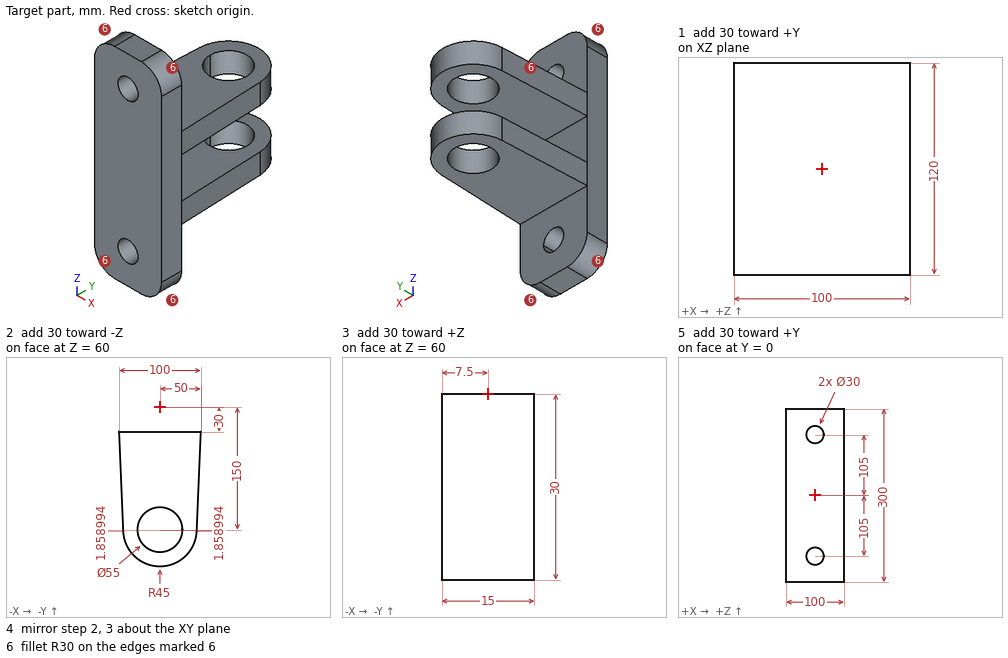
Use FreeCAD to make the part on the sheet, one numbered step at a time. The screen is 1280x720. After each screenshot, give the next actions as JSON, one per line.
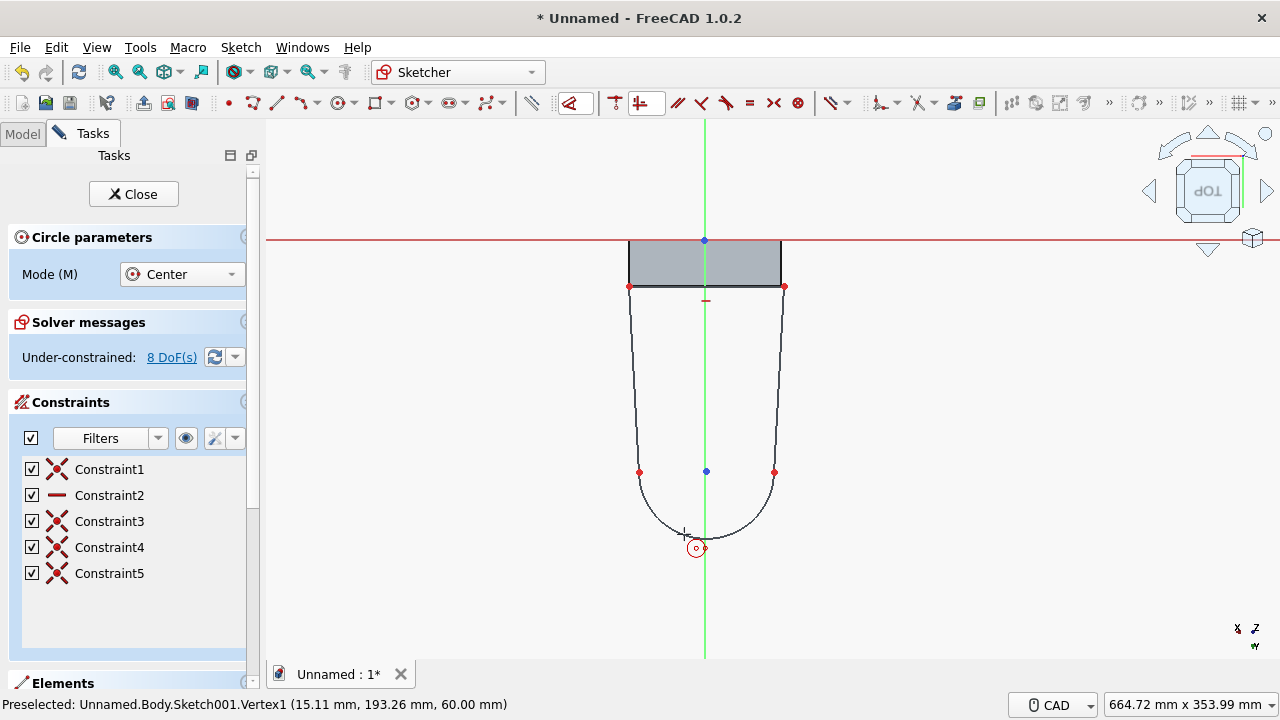
{"action": "left_click", "coordinate": [705, 469]}
{"action": "mouse_move", "coordinate": [735, 439]}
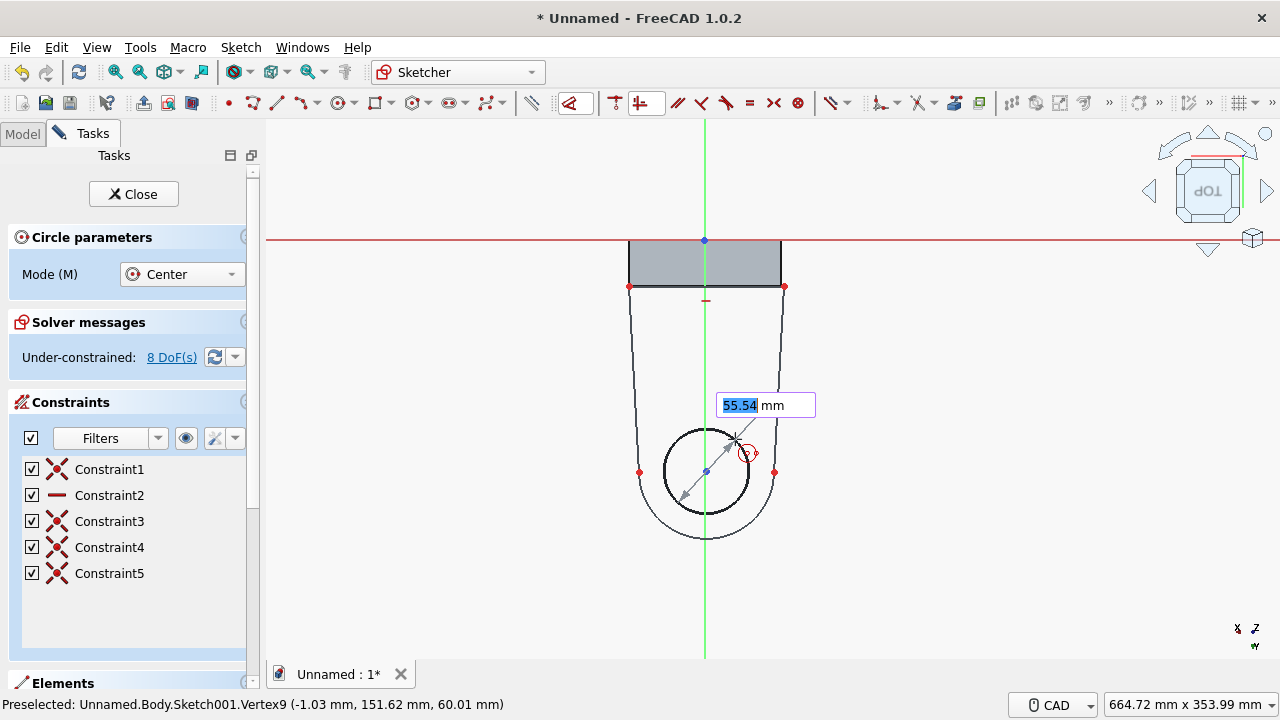
{"action": "type", "text": "55"}
{"action": "key", "text": "Return"}
{"action": "key", "text": "Escape"}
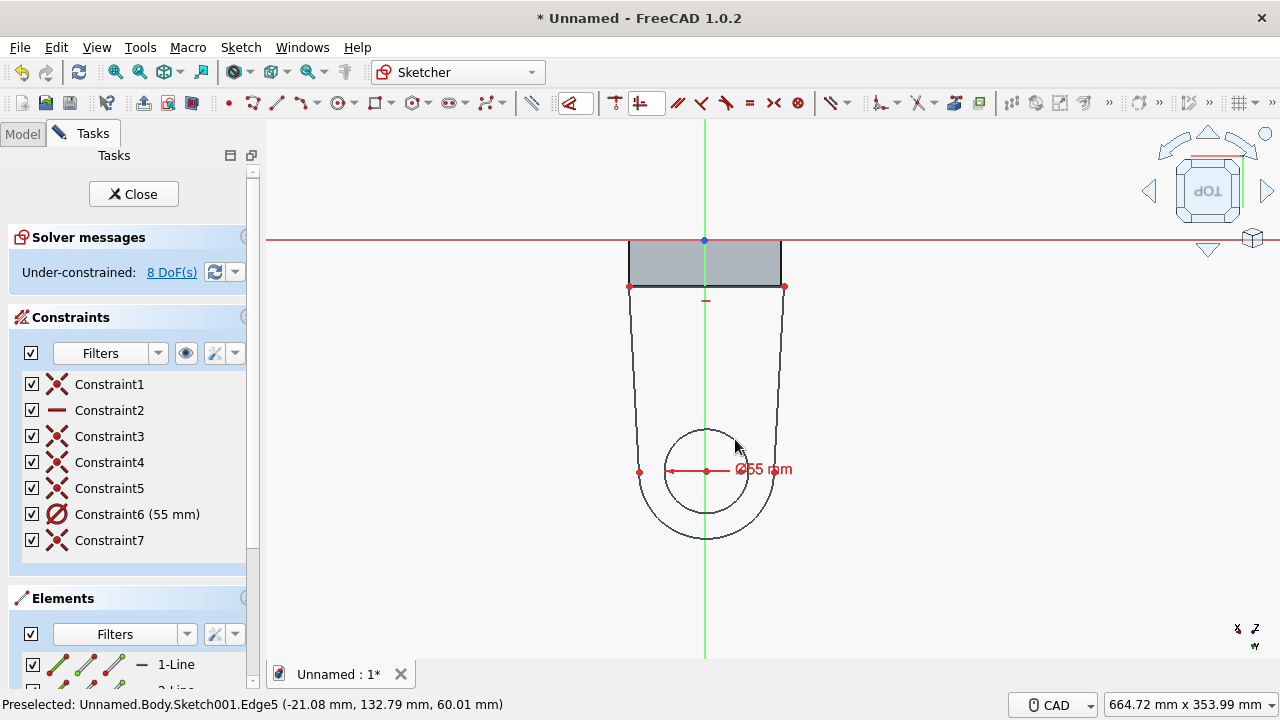
{"action": "left_click", "coordinate": [707, 471]}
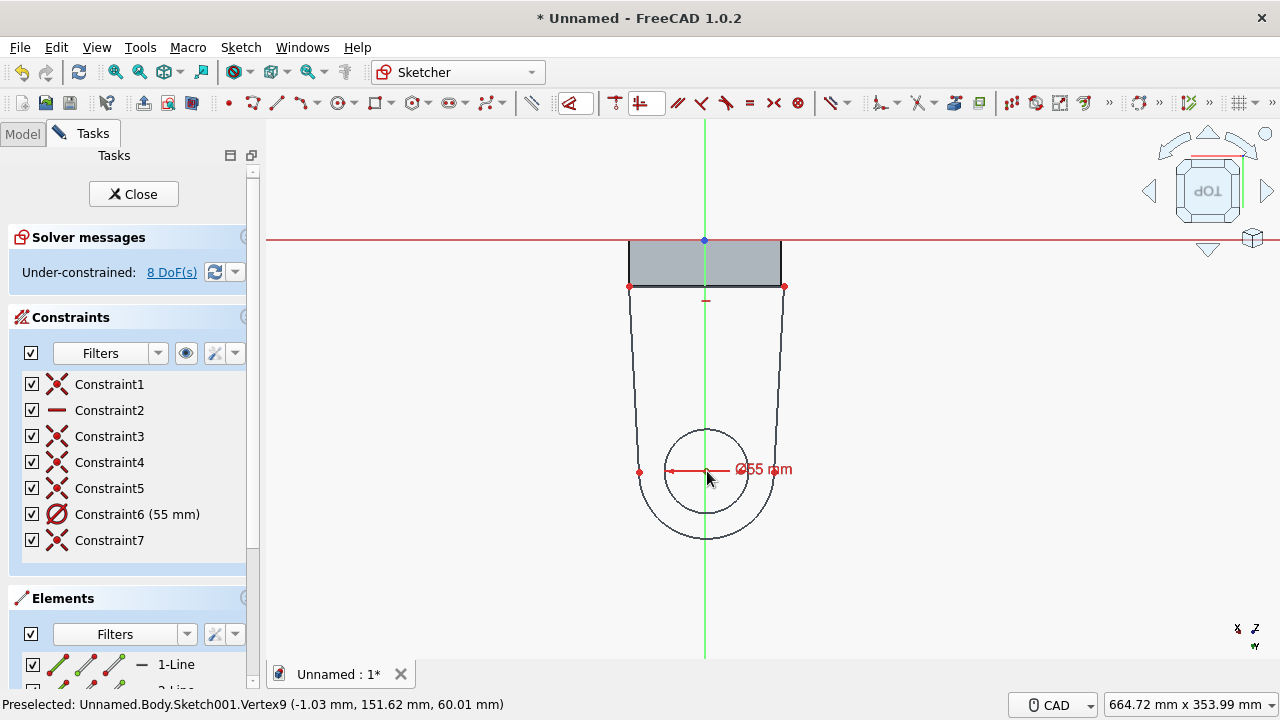
{"action": "left_click", "coordinate": [705, 596]}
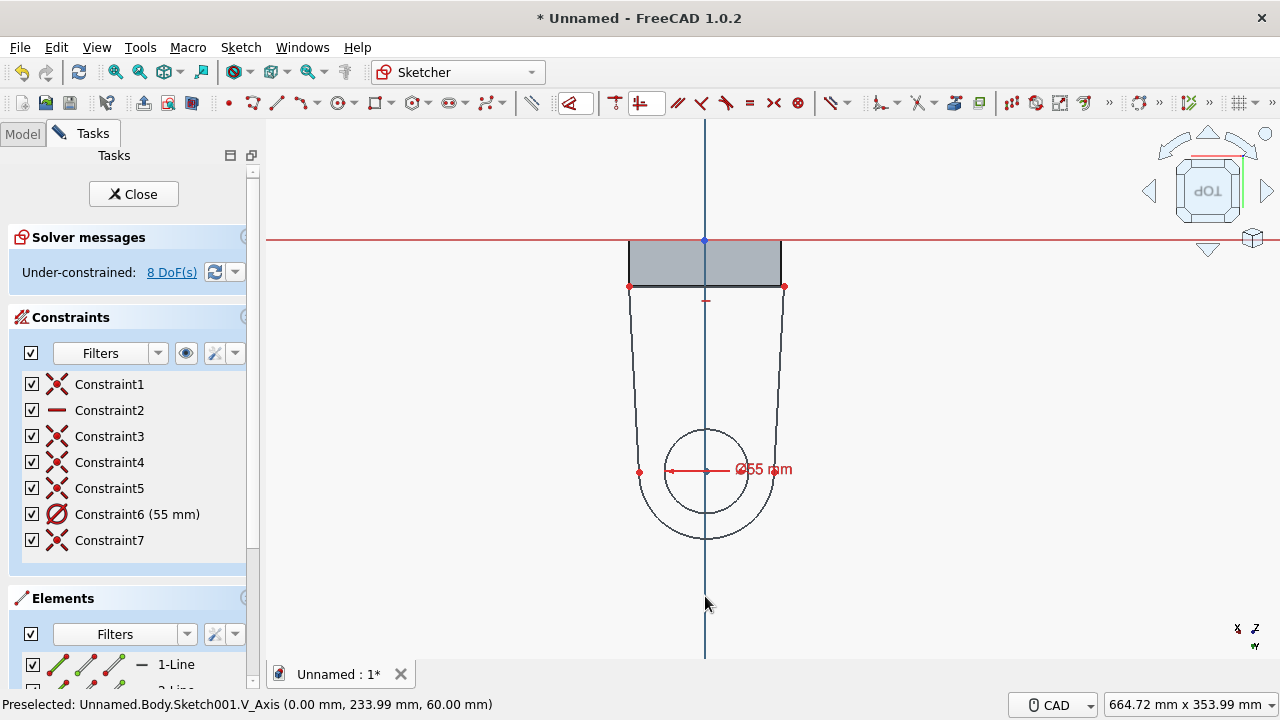
{"action": "key", "text": "c"}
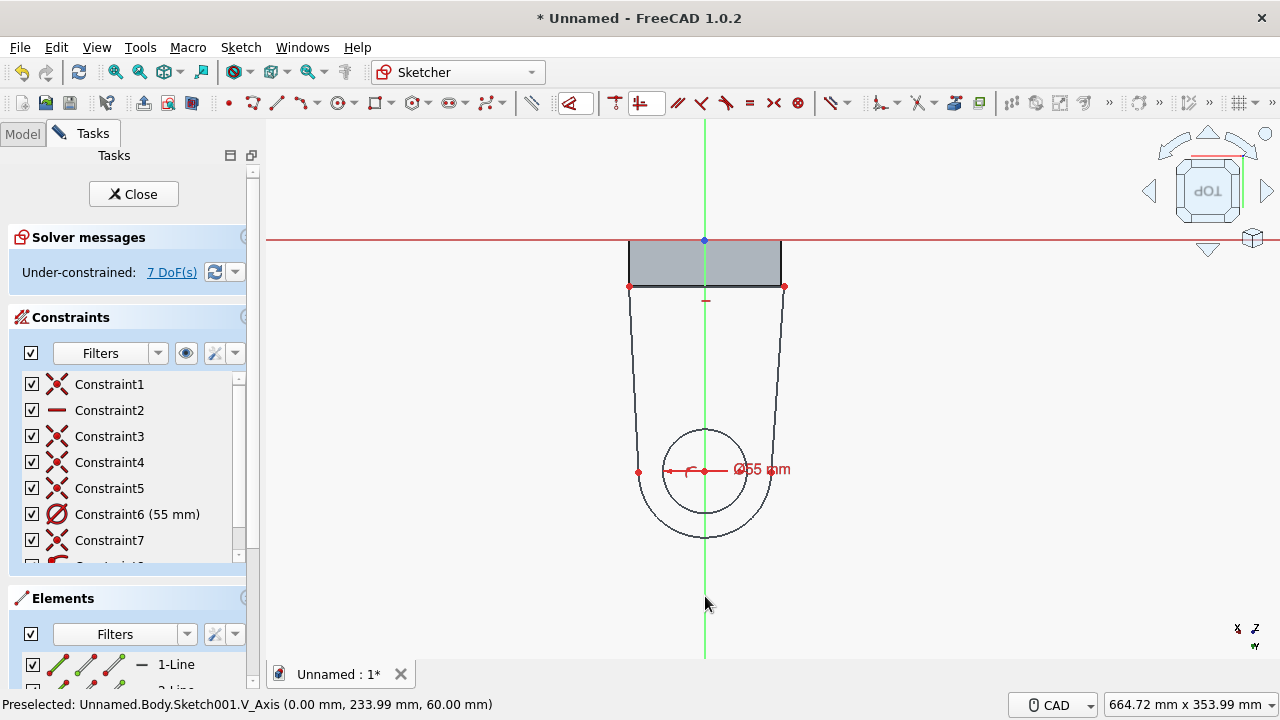
{"action": "left_click", "coordinate": [666, 525]}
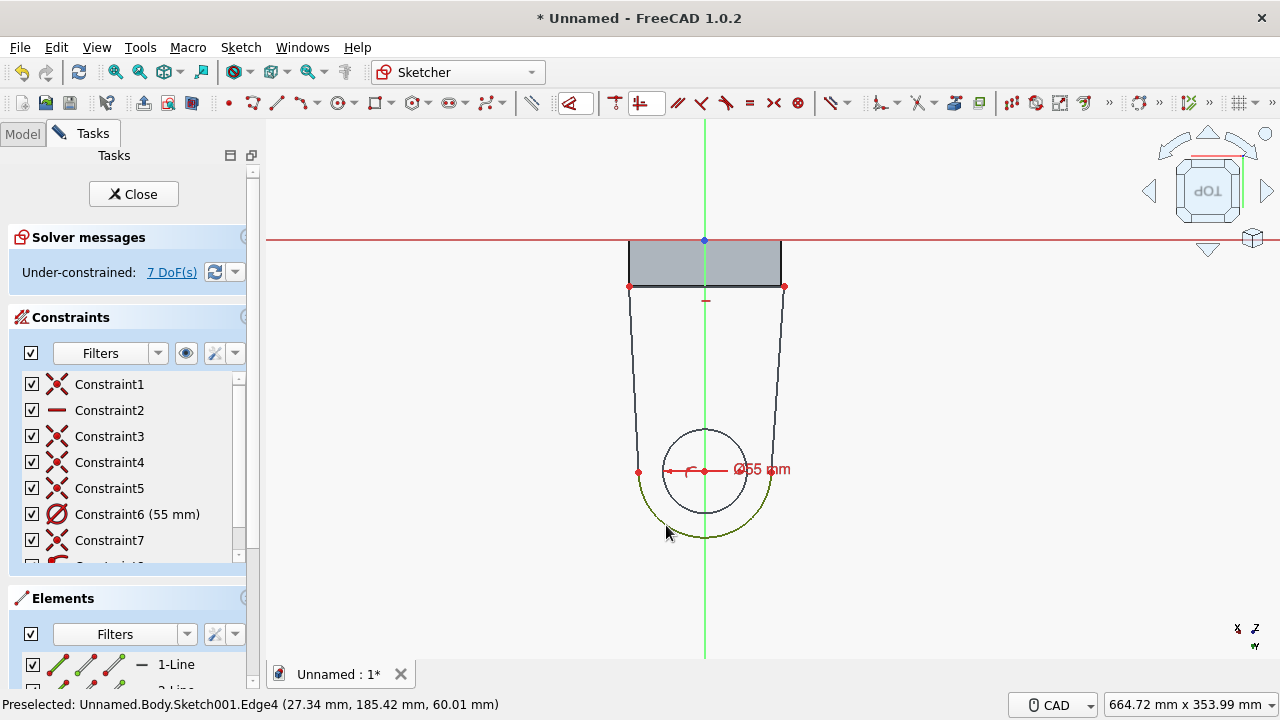
{"action": "key", "text": "k r"}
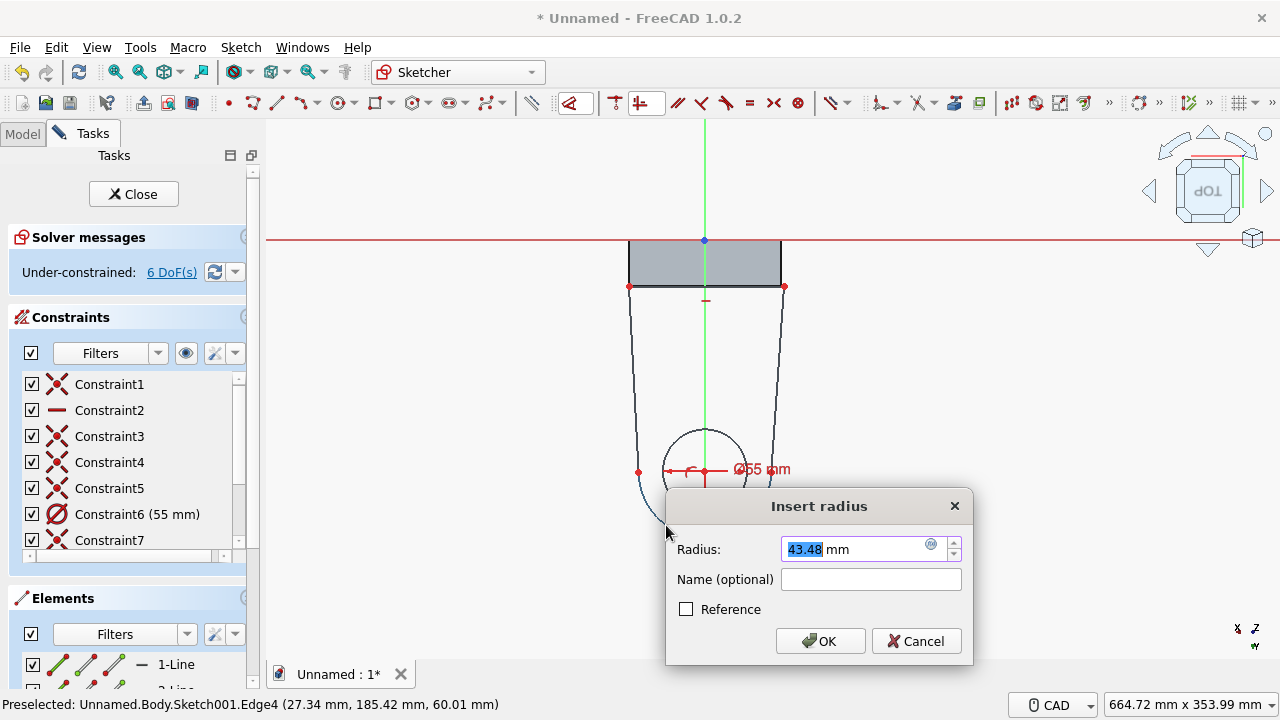
{"action": "type", "text": "45"}
{"action": "key", "text": "Return"}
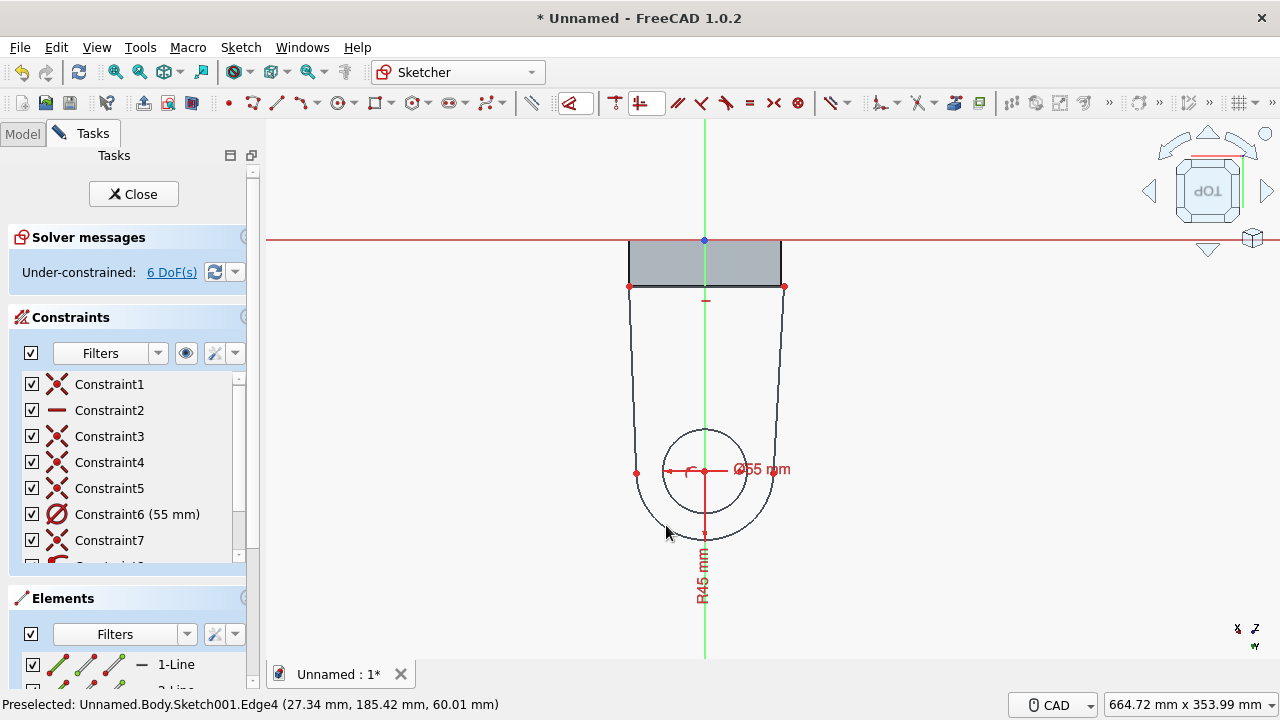
{"action": "left_click", "coordinate": [737, 287]}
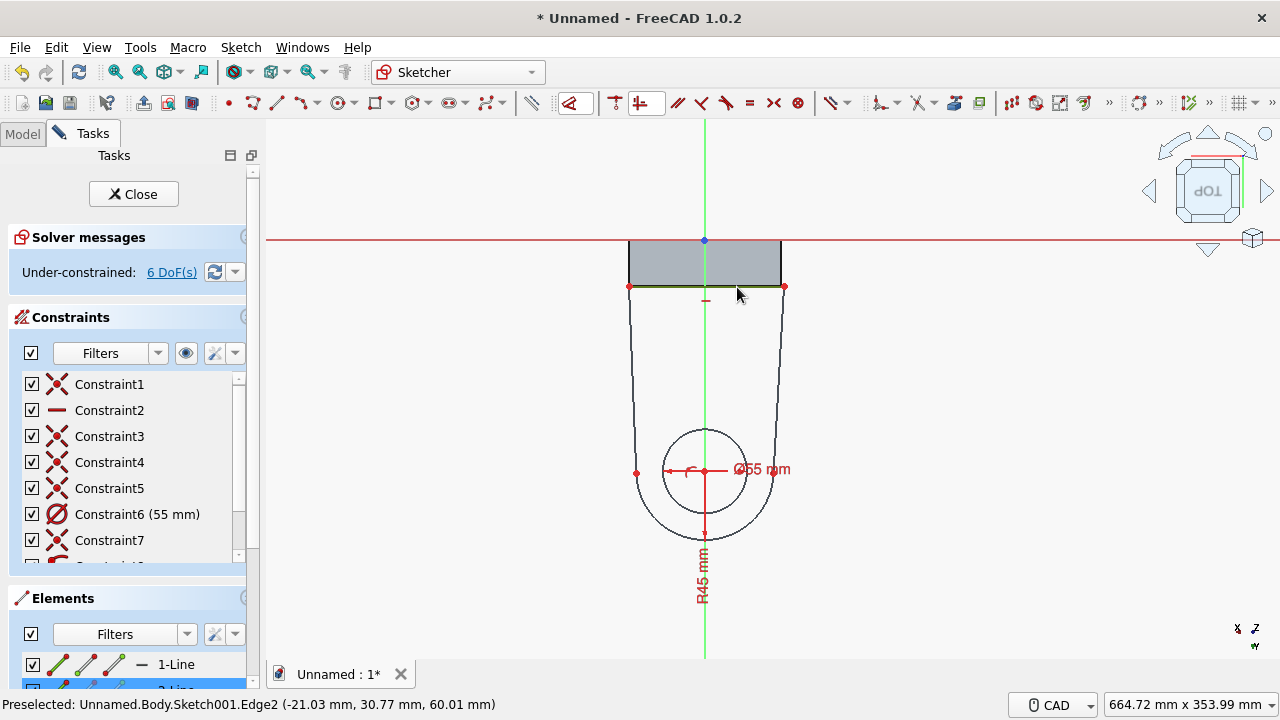
{"action": "key", "text": "l"}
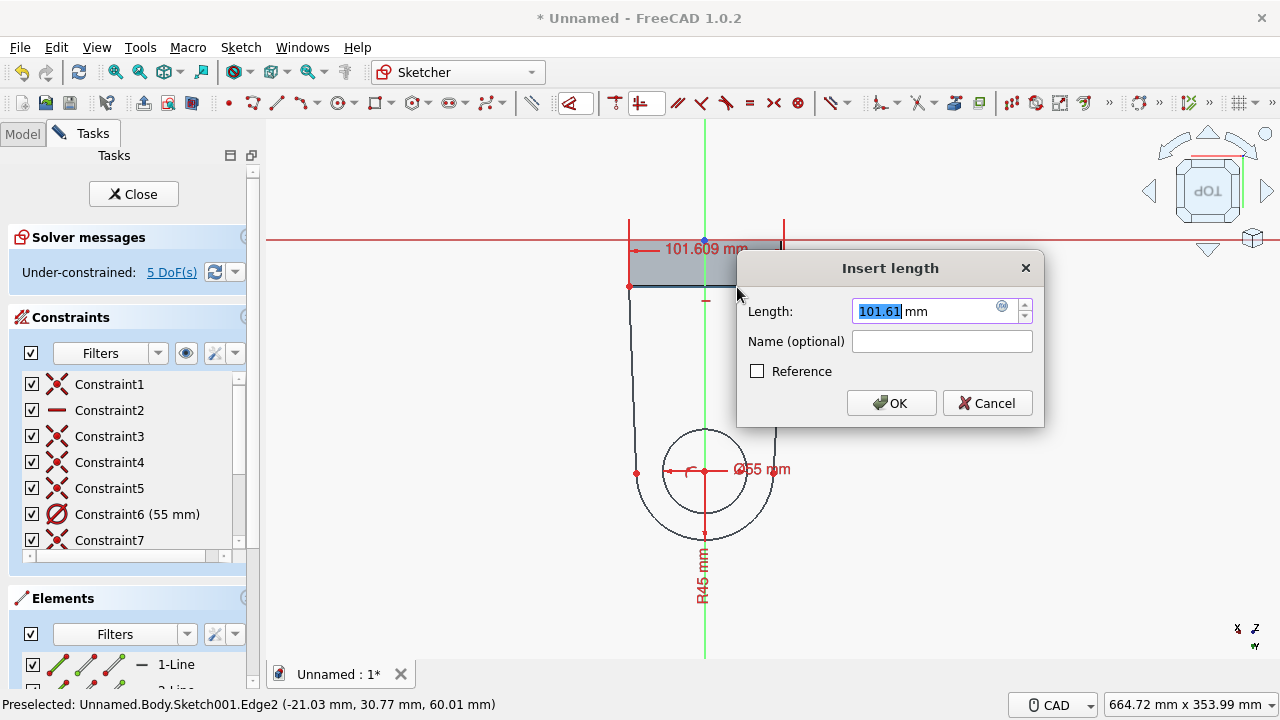
{"action": "type", "text": "100"}
{"action": "key", "text": "Return"}